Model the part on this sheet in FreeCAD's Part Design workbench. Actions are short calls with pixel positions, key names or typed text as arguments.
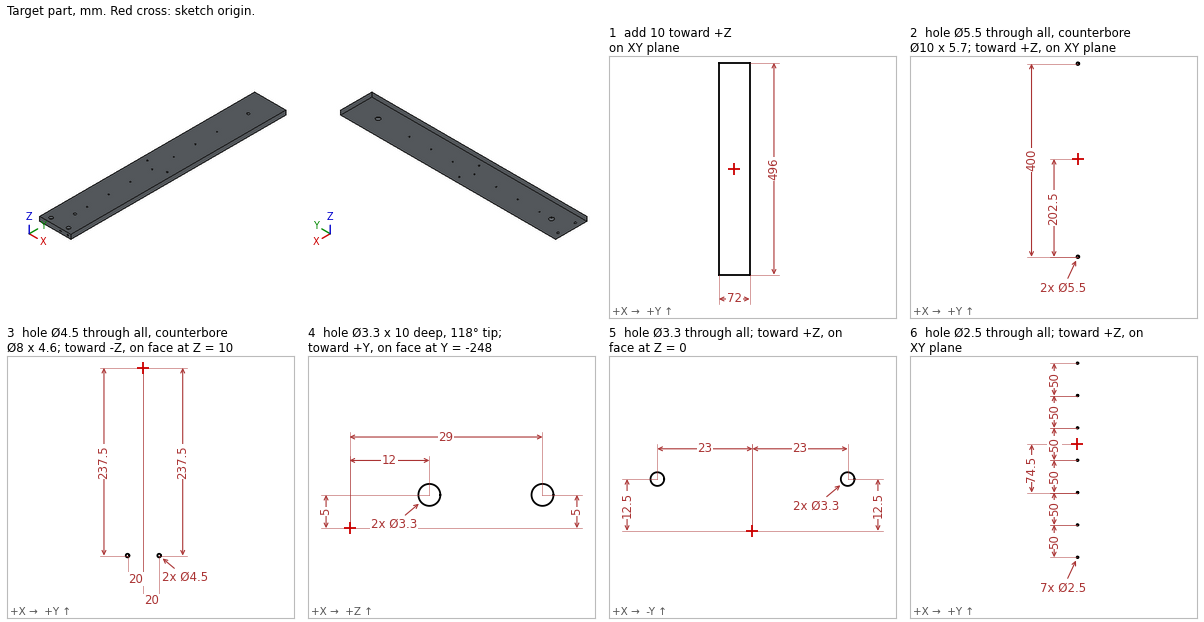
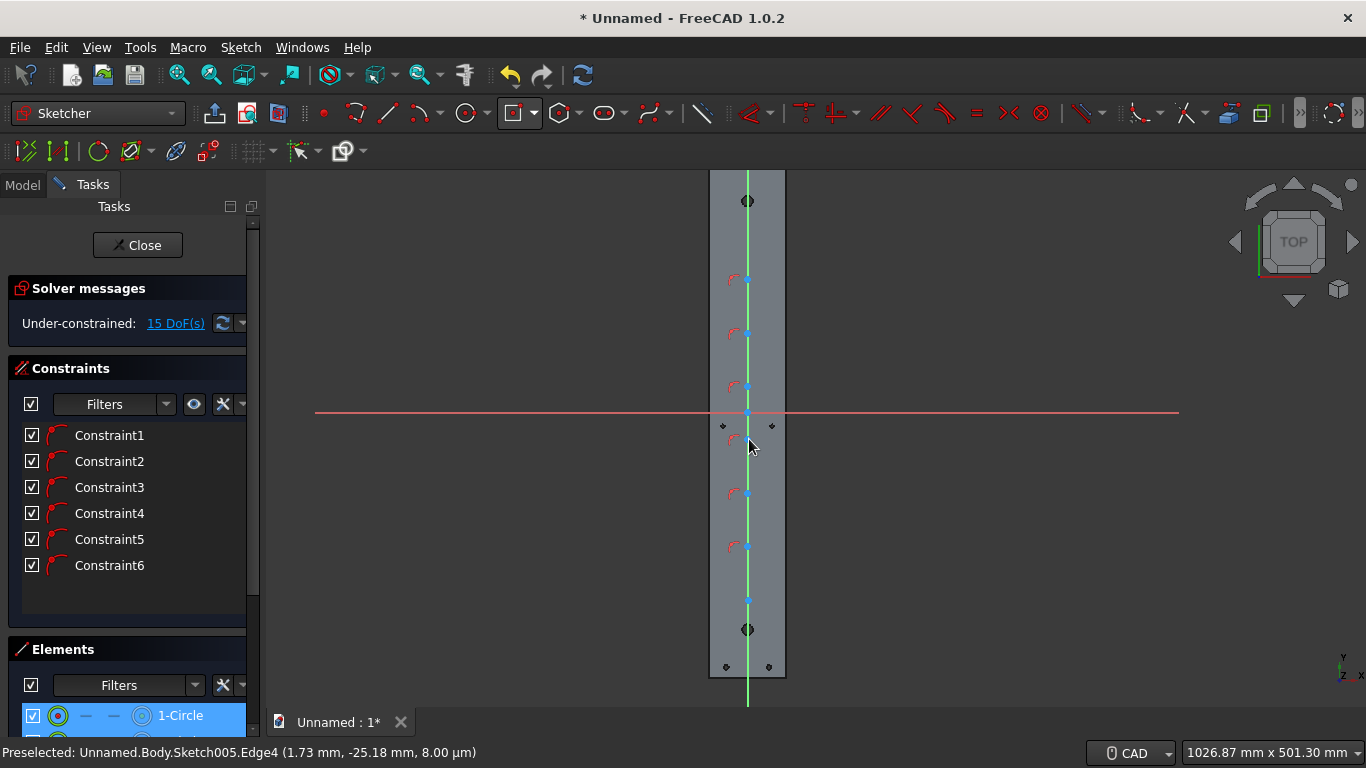
scroll(749, 385, up, 13)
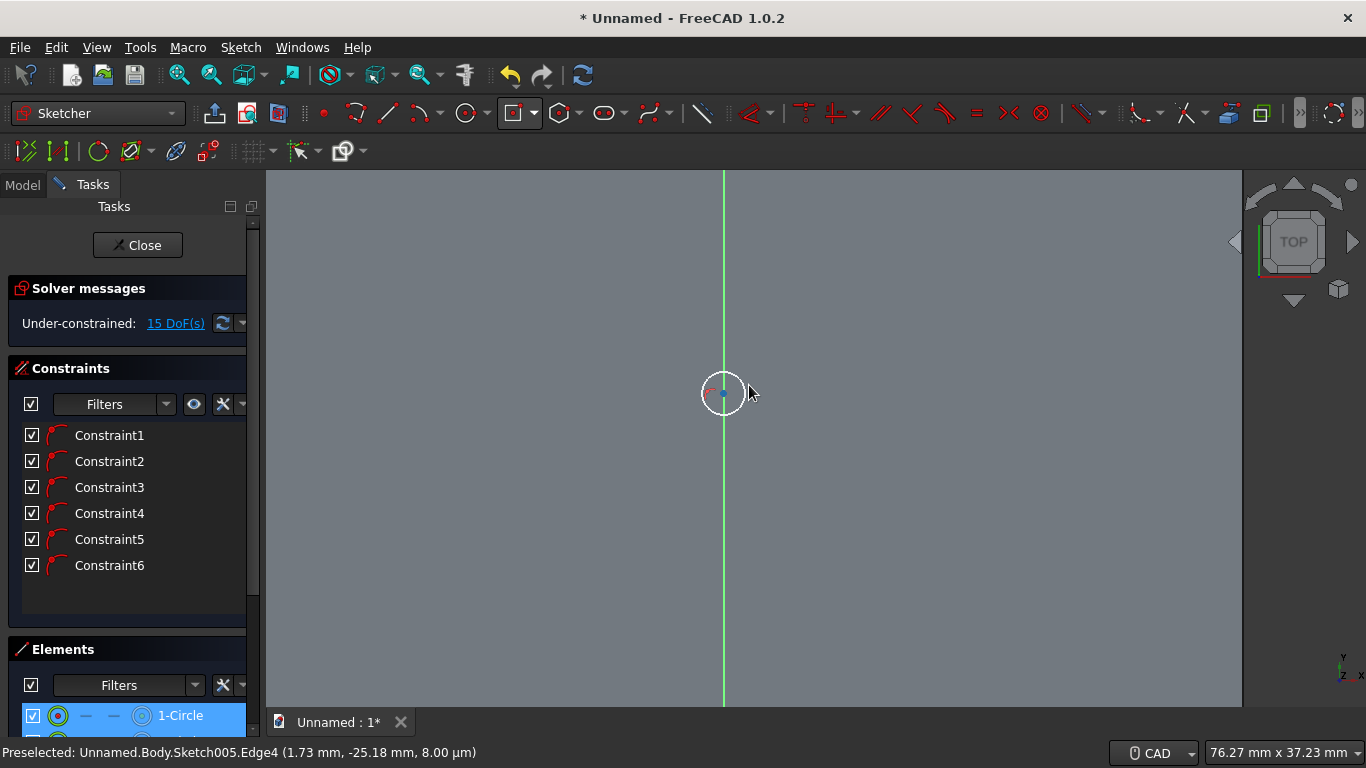
click(739, 378)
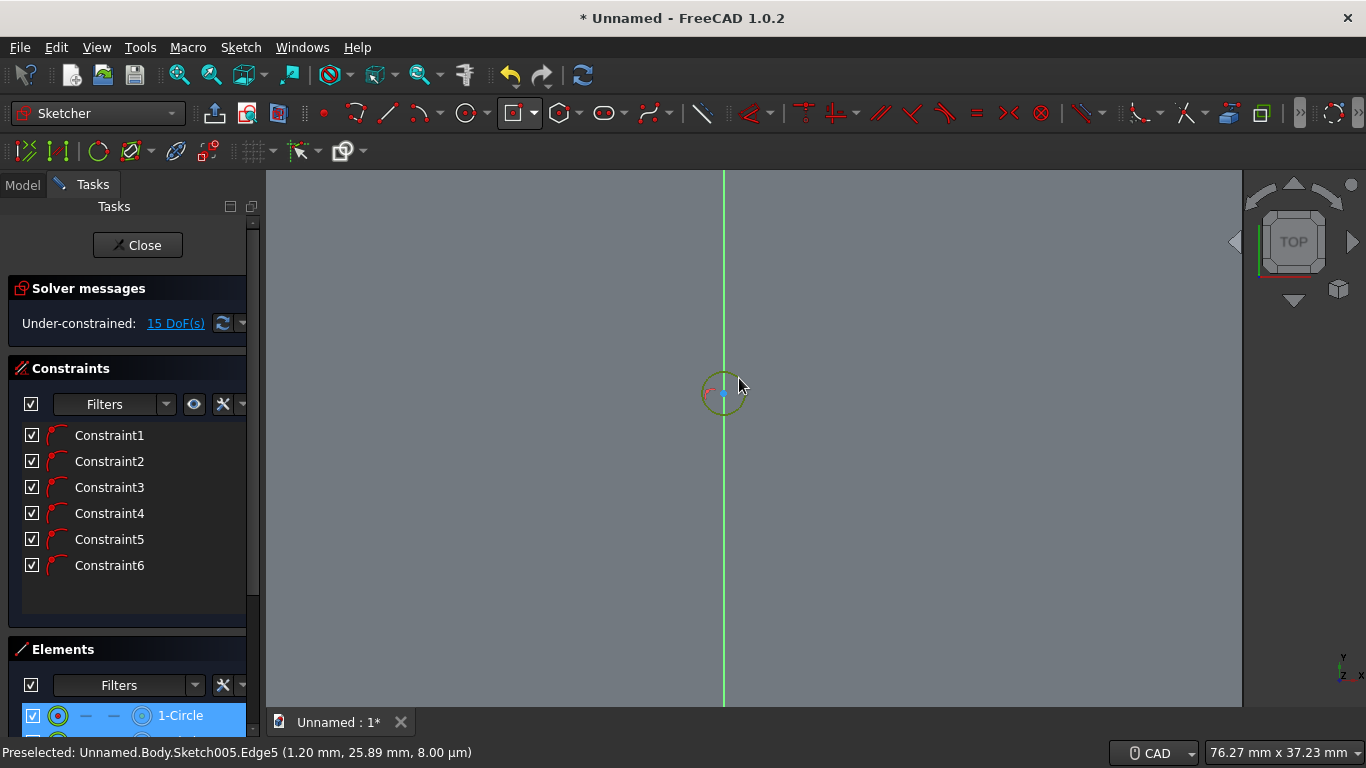
scroll(749, 385, down, 13)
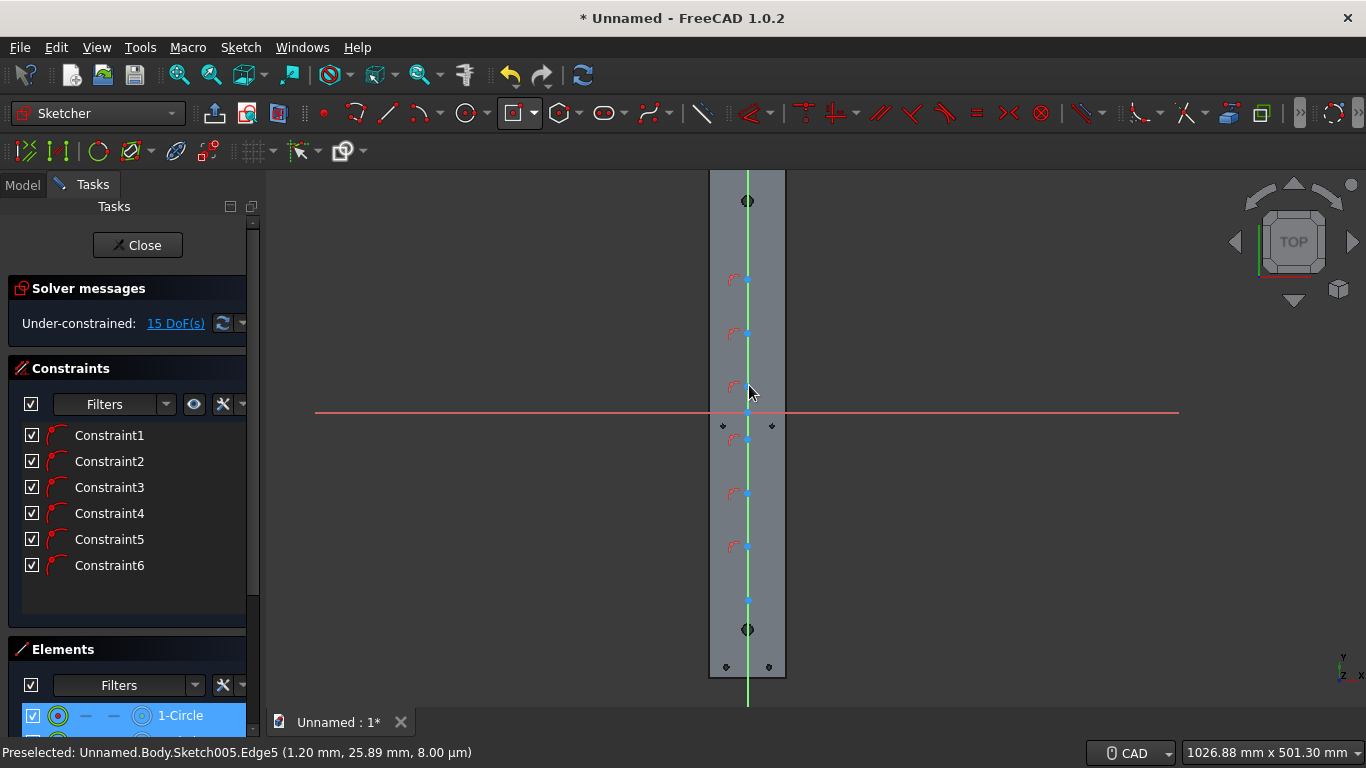
scroll(749, 332, up, 12)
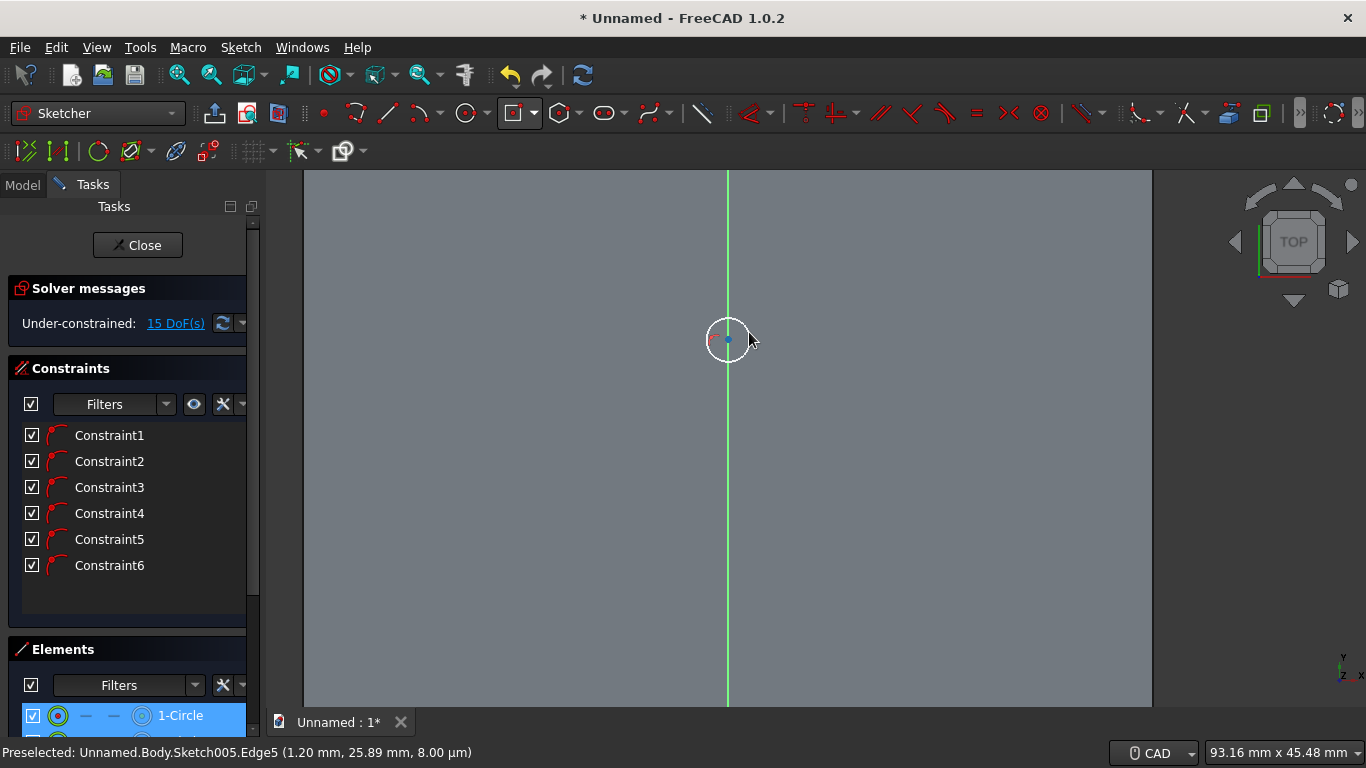
click(744, 325)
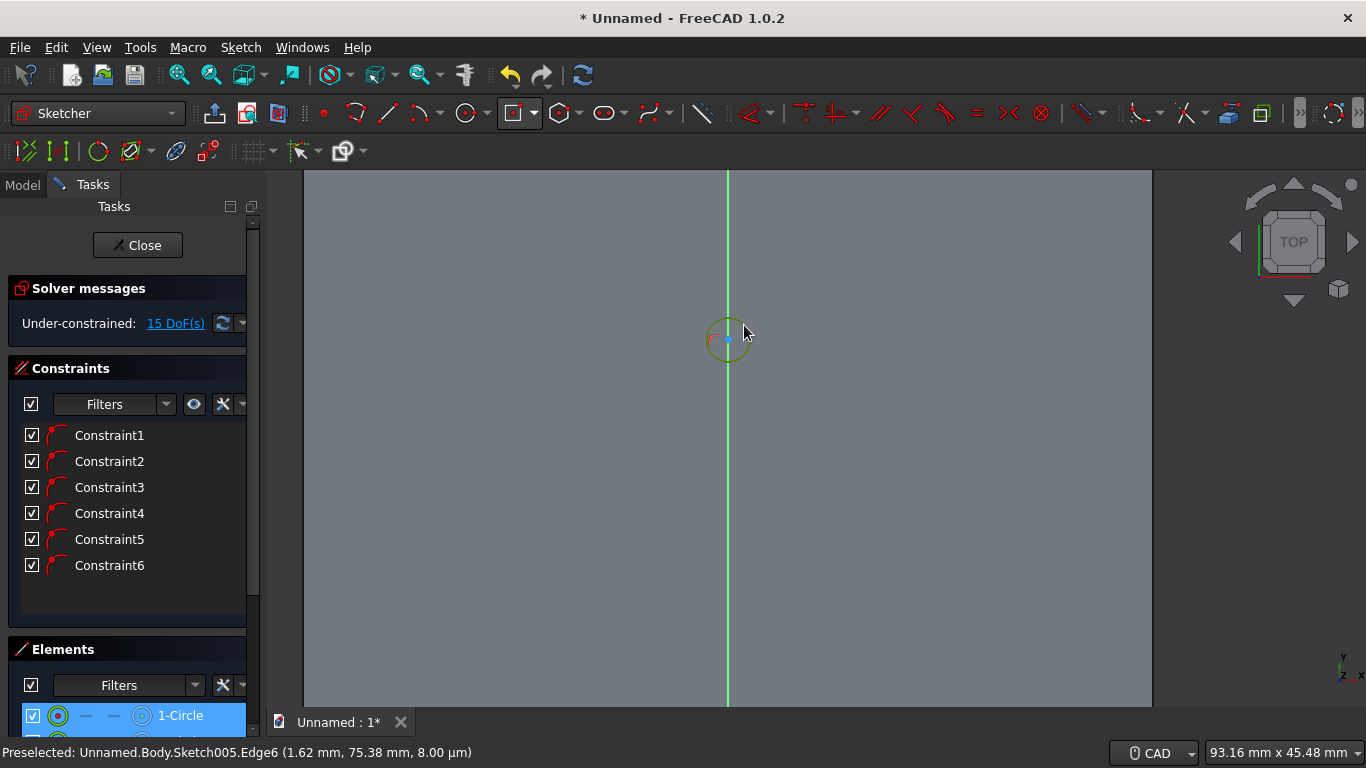
scroll(749, 332, down, 12)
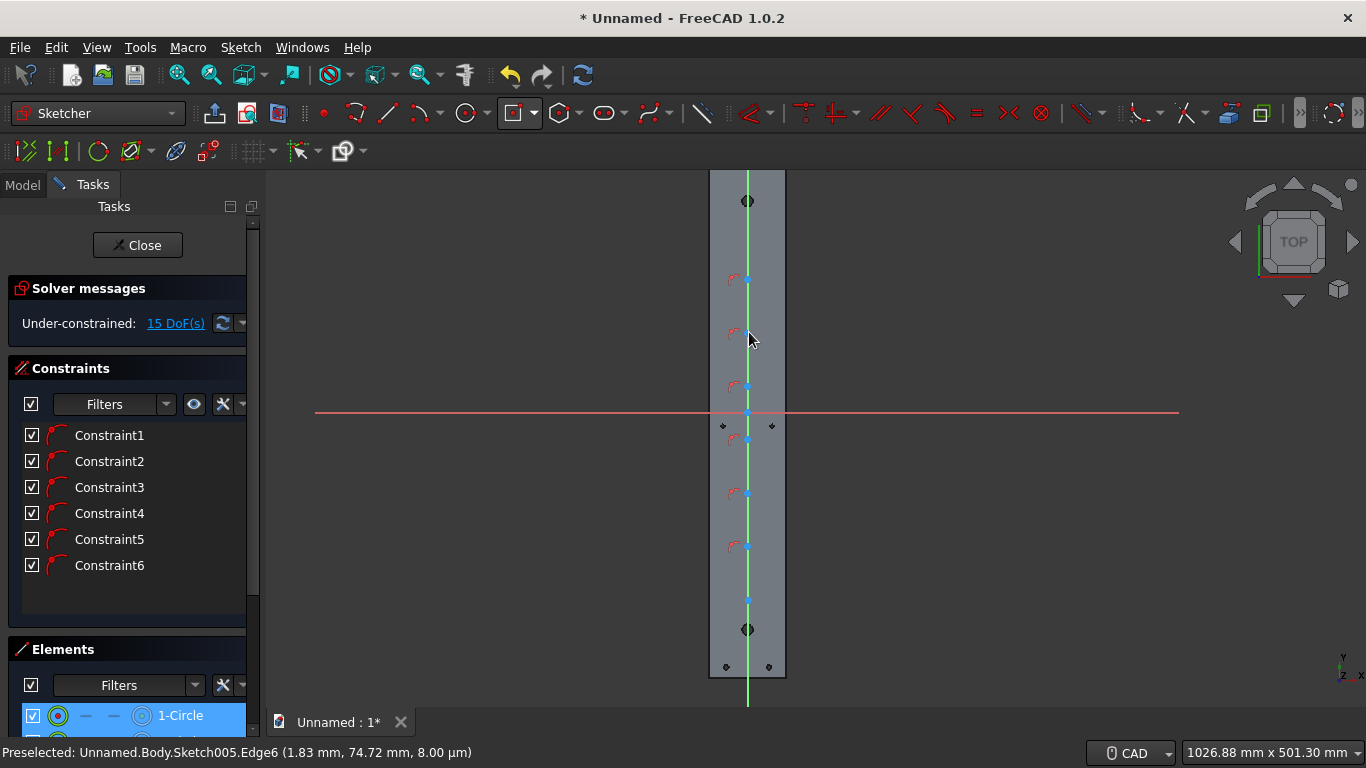
scroll(749, 278, up, 13)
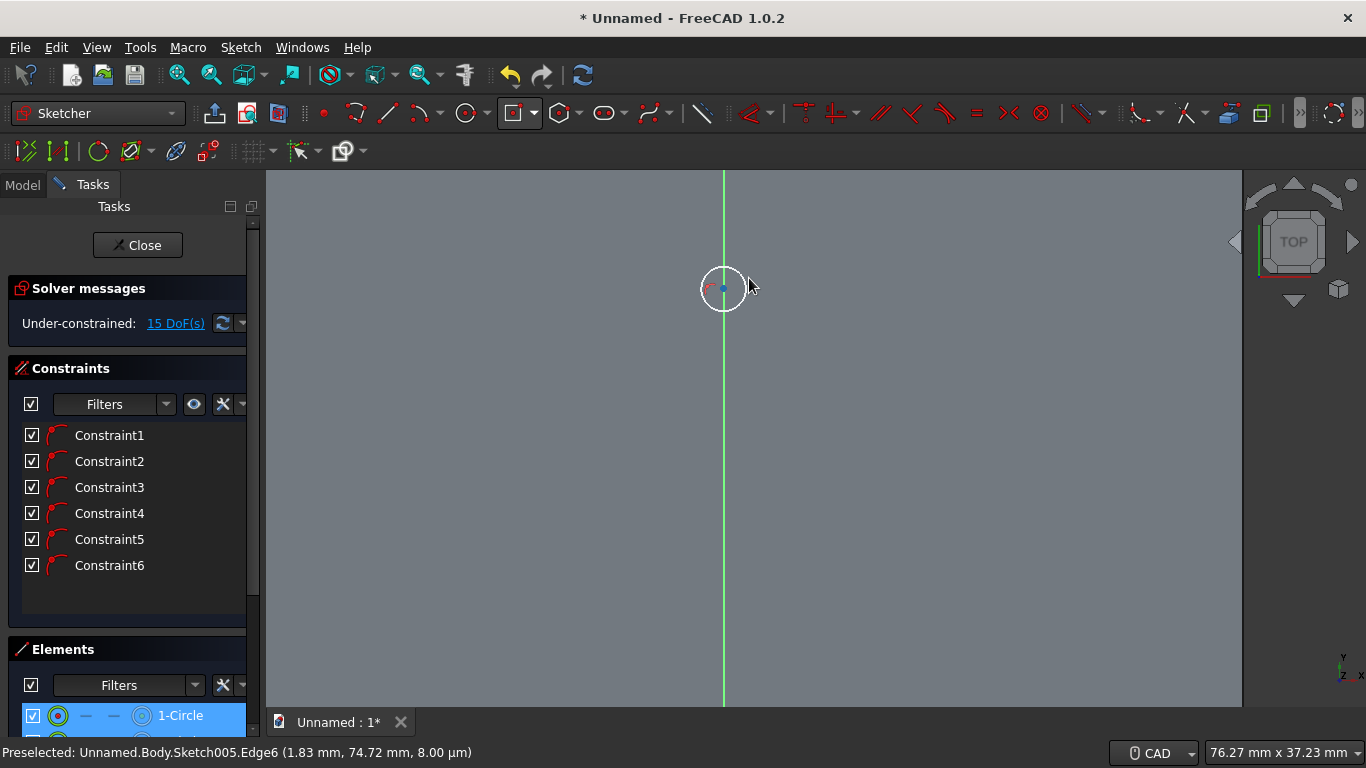
click(739, 273)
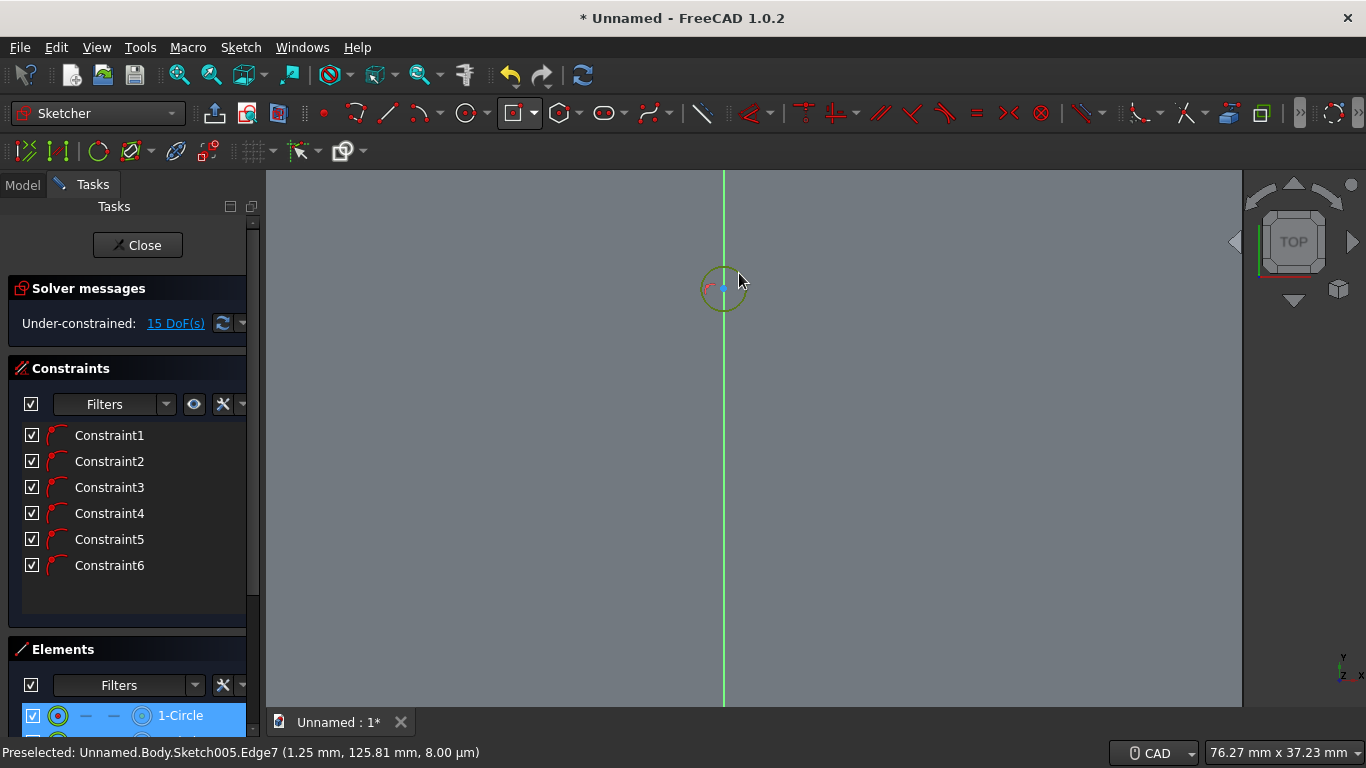
click(978, 114)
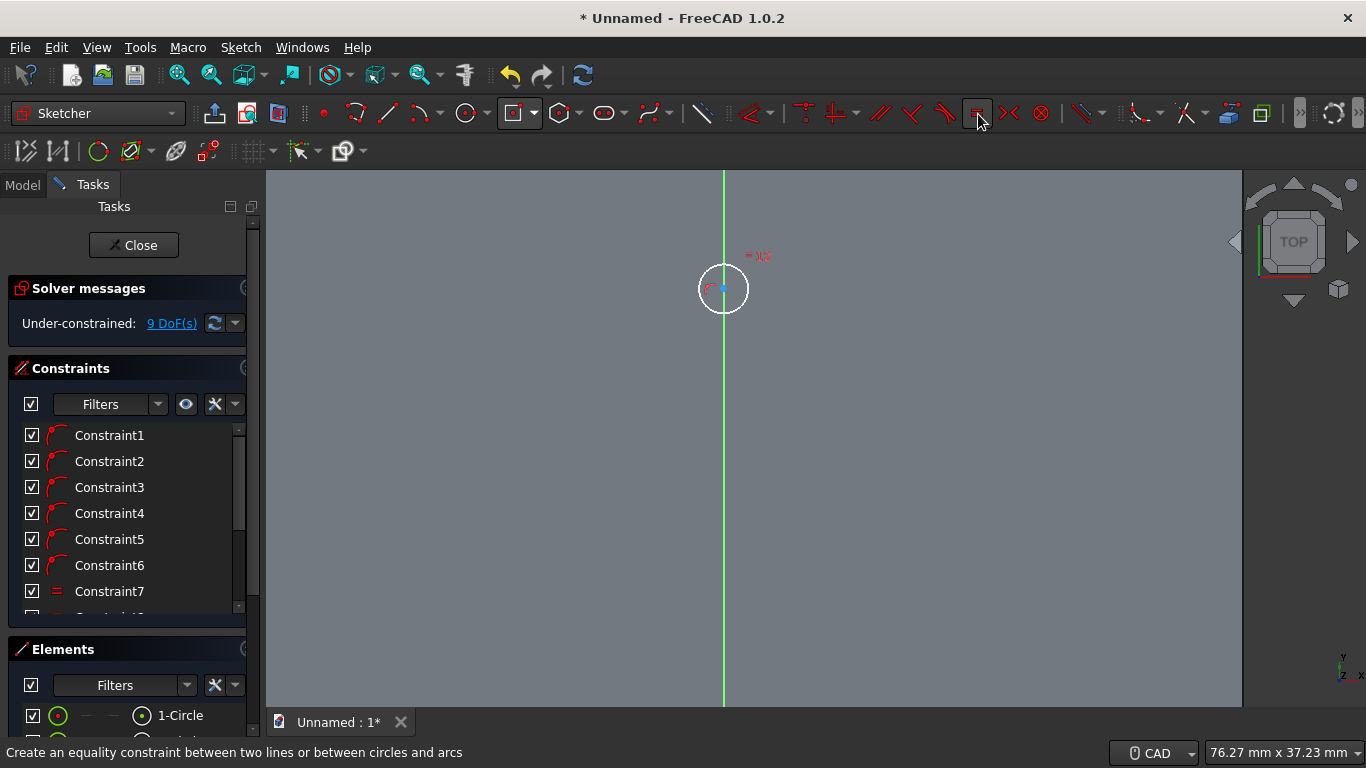
scroll(749, 278, down, 13)